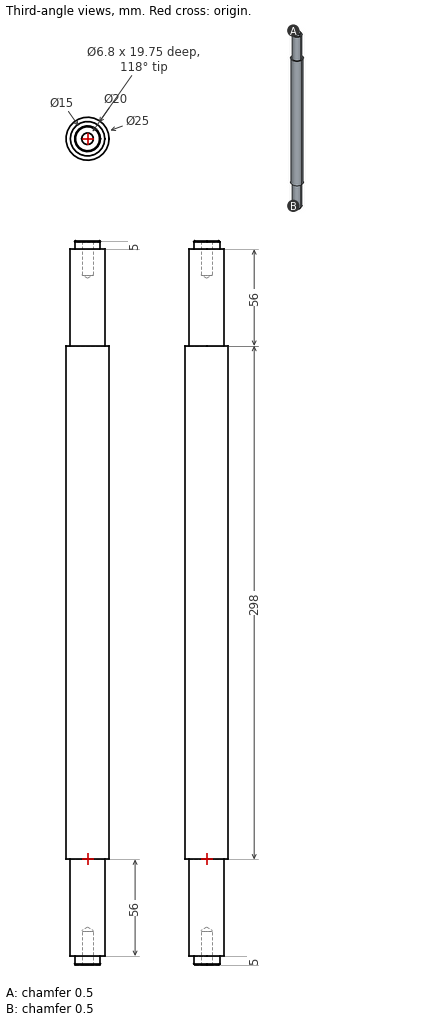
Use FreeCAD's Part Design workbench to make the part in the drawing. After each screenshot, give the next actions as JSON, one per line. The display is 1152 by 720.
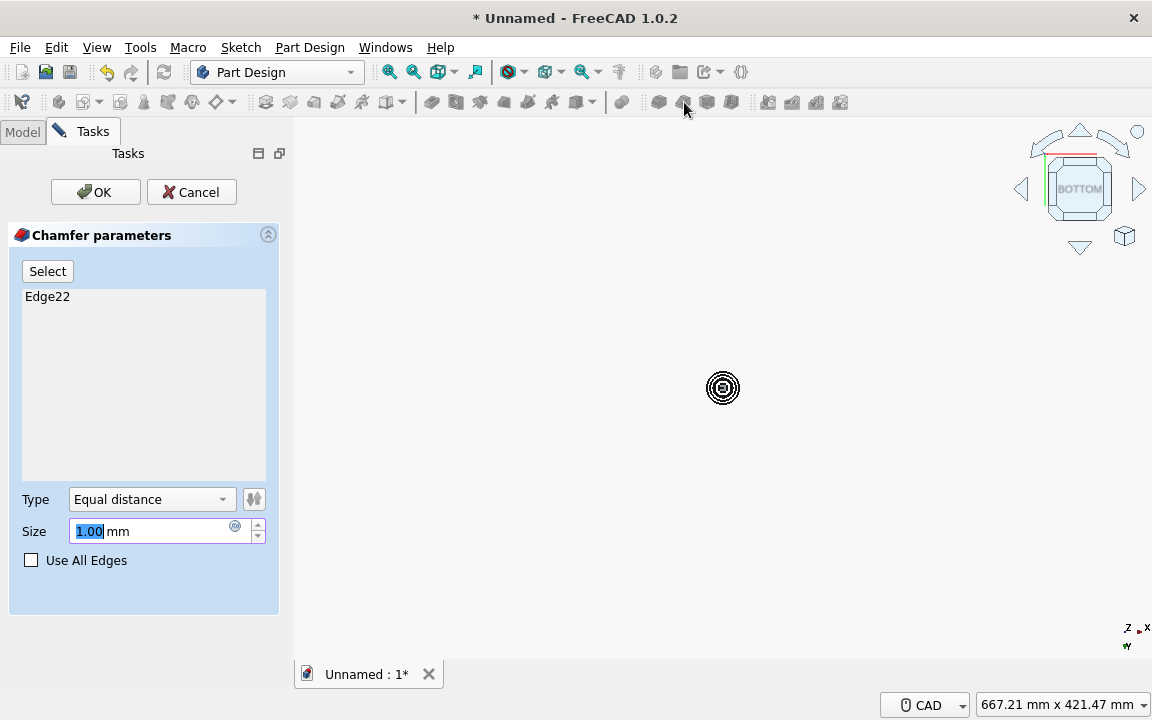
{"action": "type", "text": "0.5"}
{"action": "key", "text": "Tab"}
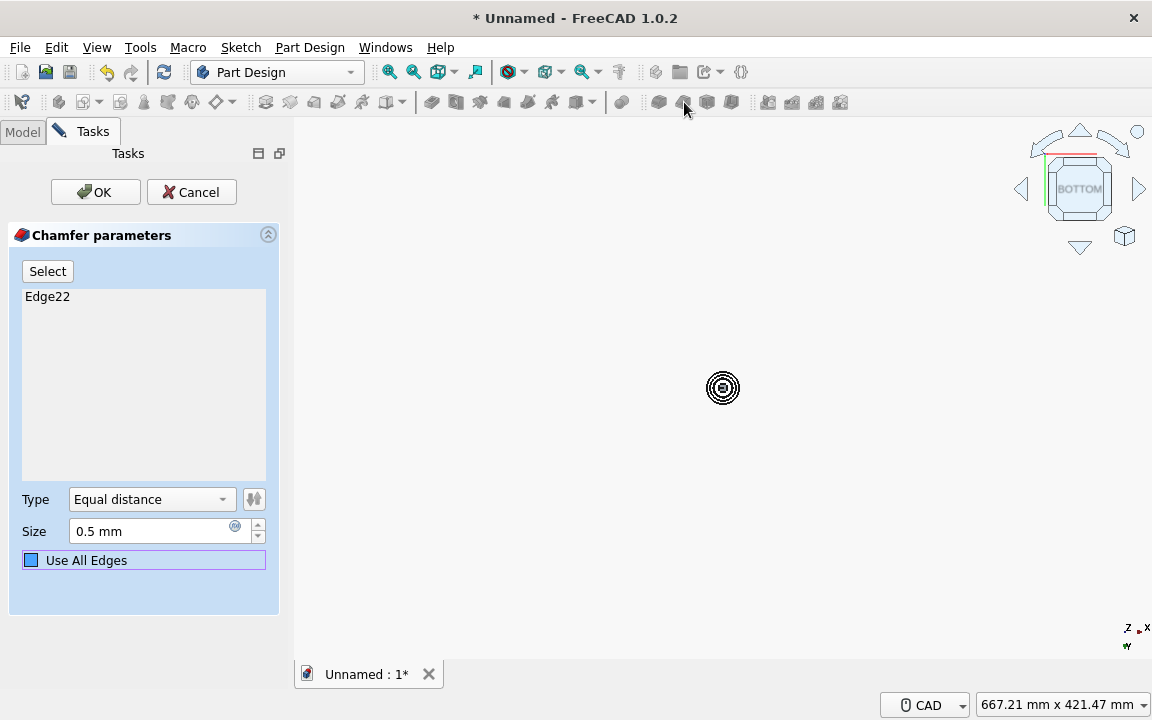
{"action": "left_click", "coordinate": [96, 192]}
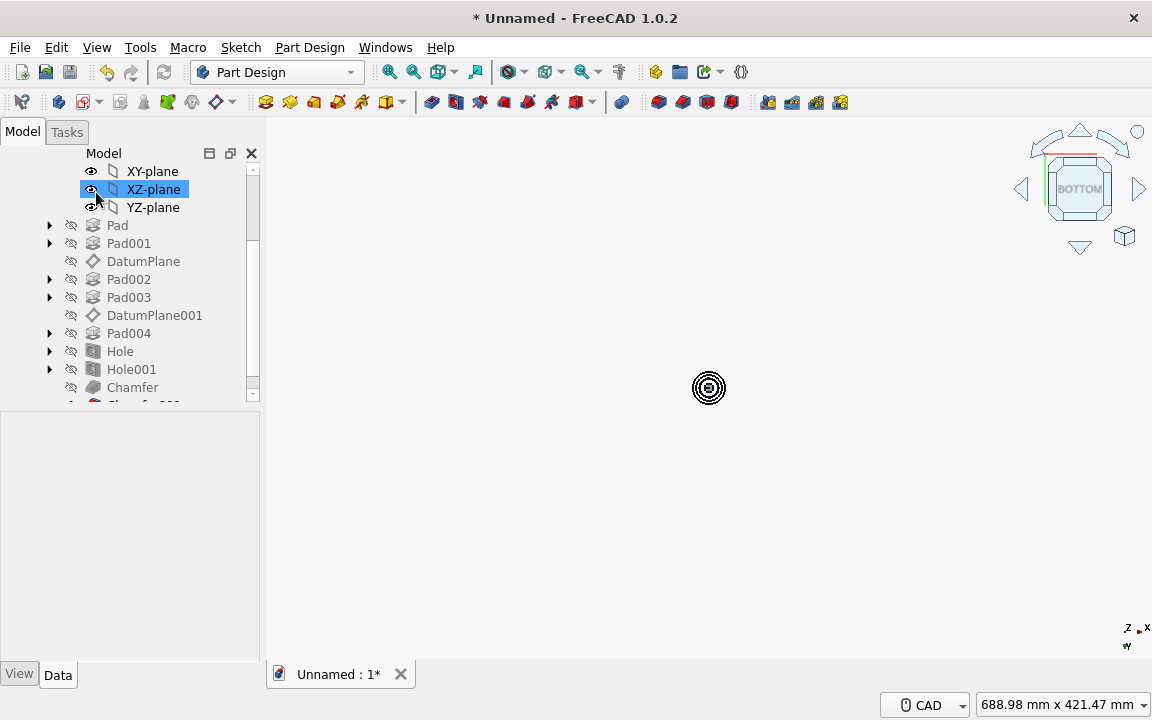
{"action": "key", "text": "0"}